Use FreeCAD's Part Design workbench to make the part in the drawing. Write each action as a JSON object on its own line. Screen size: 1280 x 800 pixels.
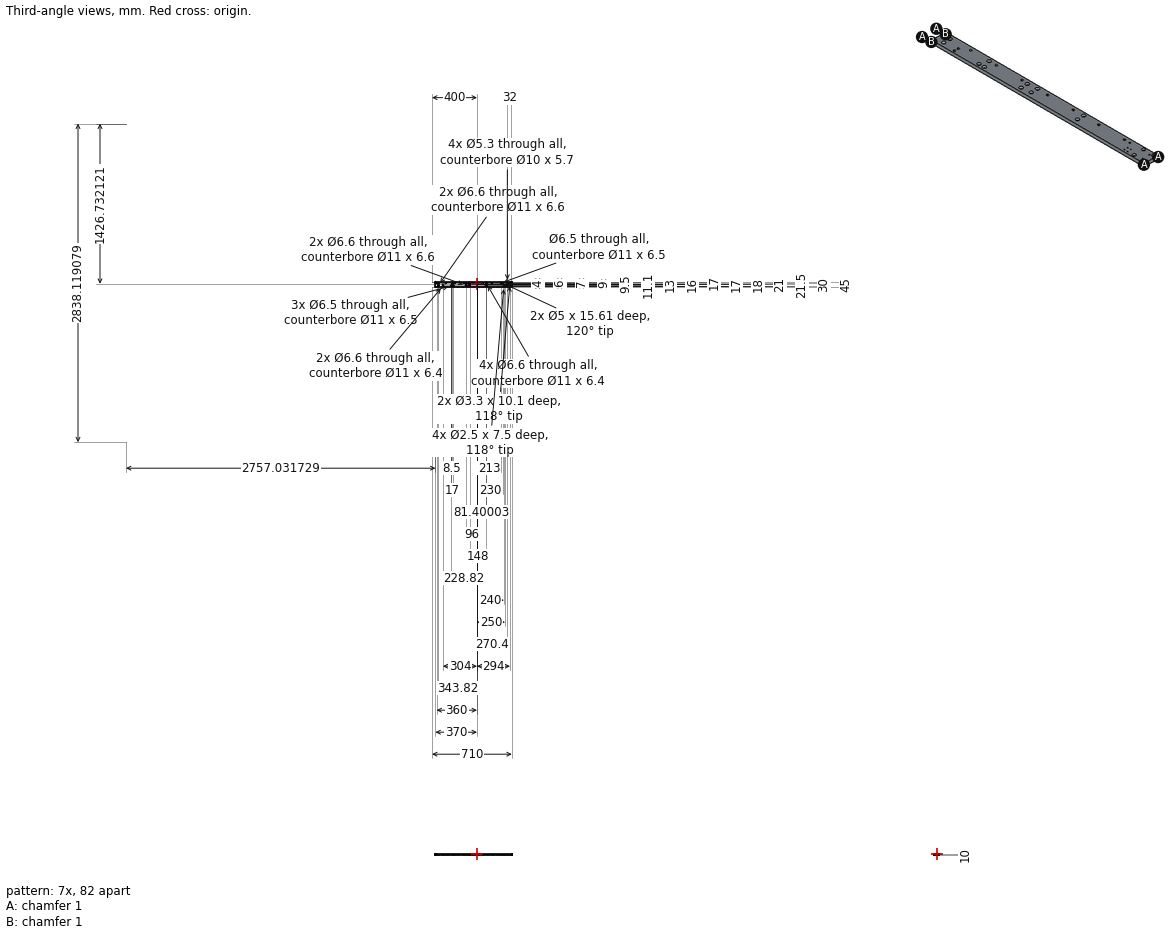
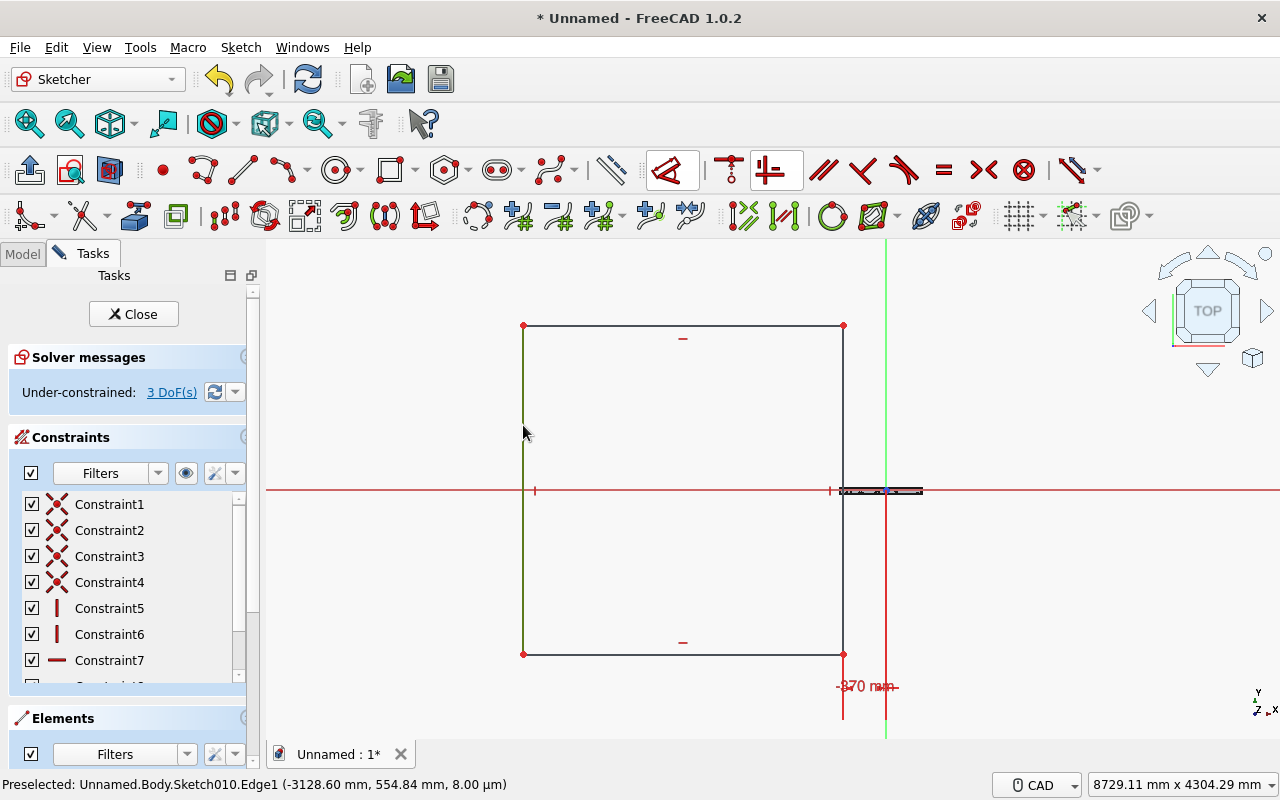
{"action": "left_click", "coordinate": [694, 170]}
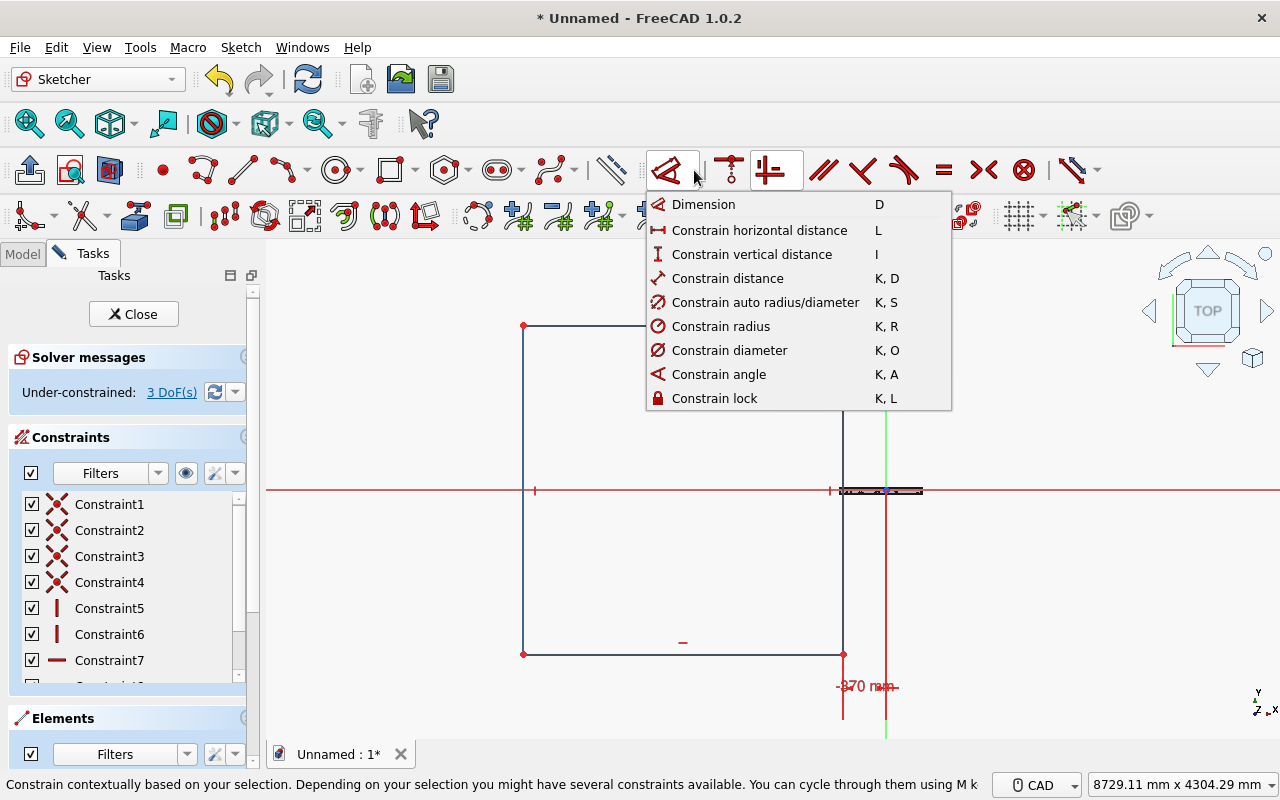
{"action": "left_click", "coordinate": [799, 254]}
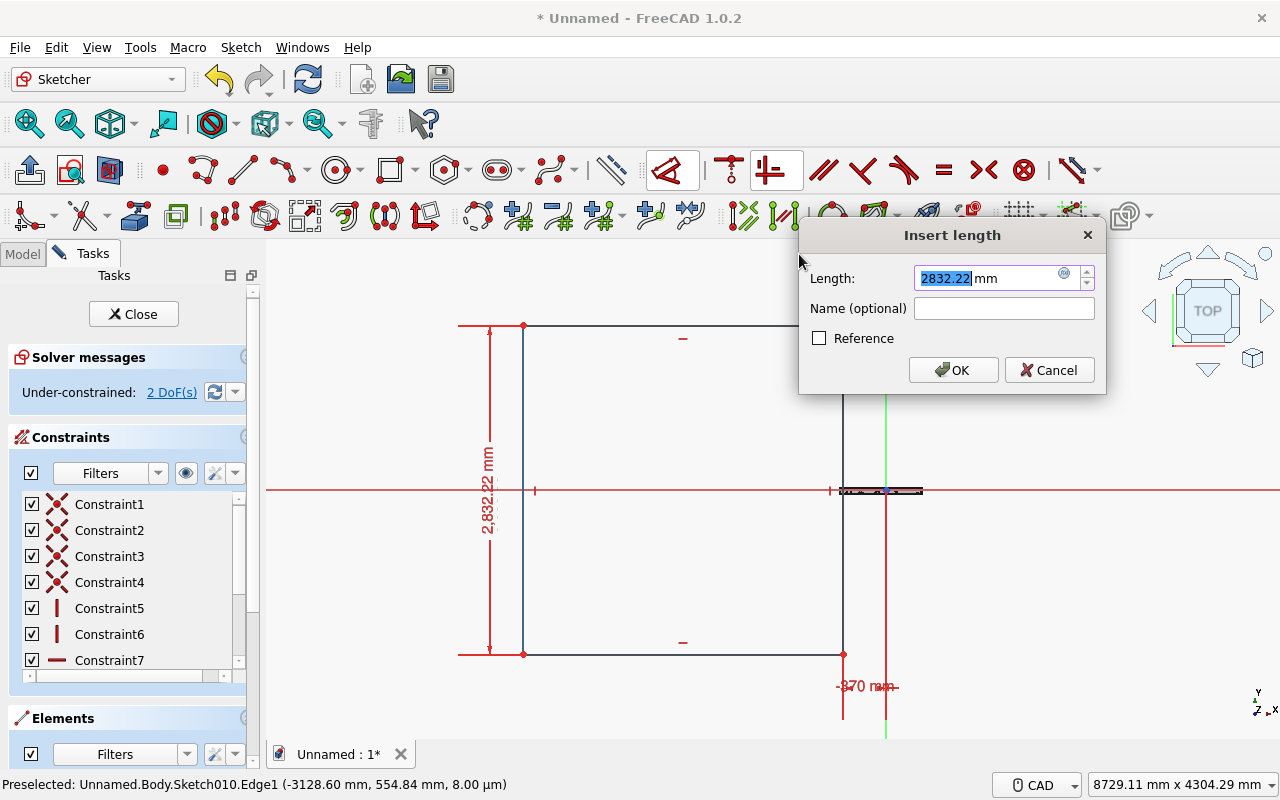
{"action": "type", "text": "2838.119079"}
{"action": "key", "text": "Return"}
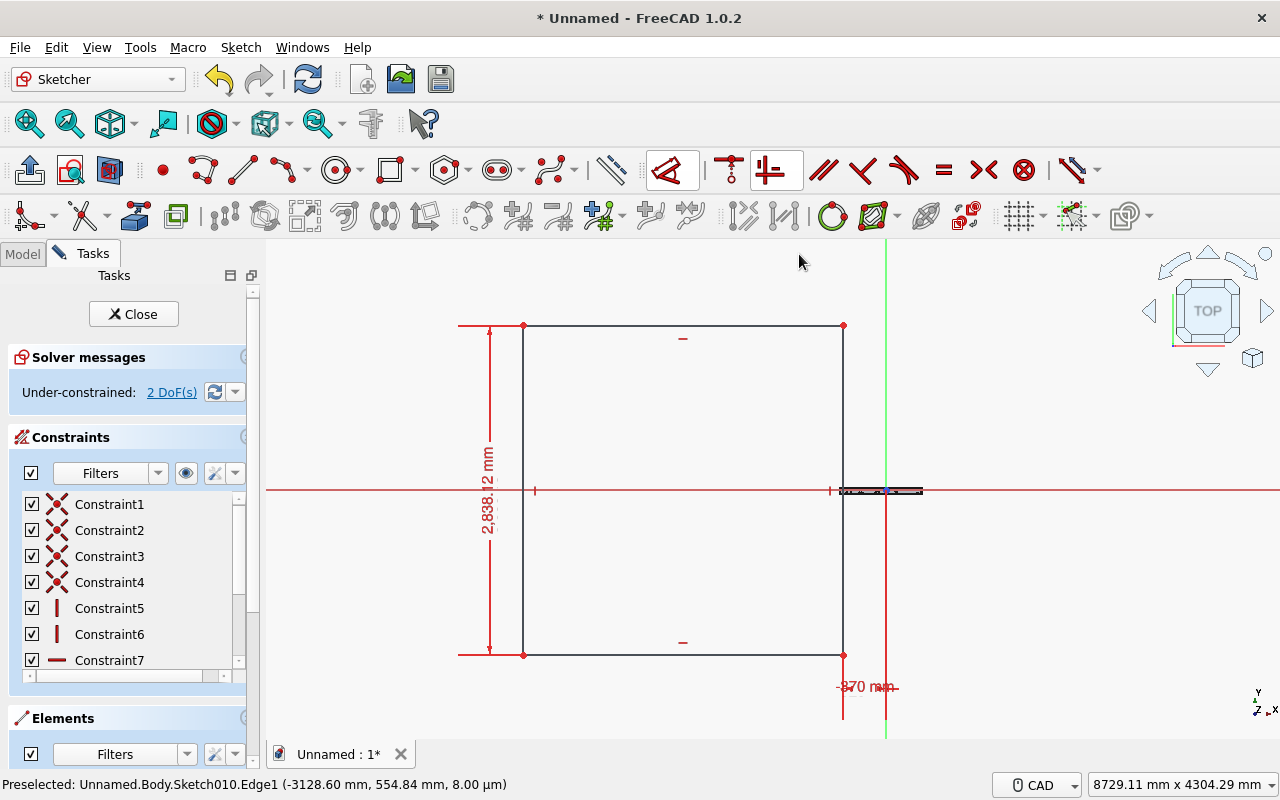
{"action": "left_click", "coordinate": [619, 655]}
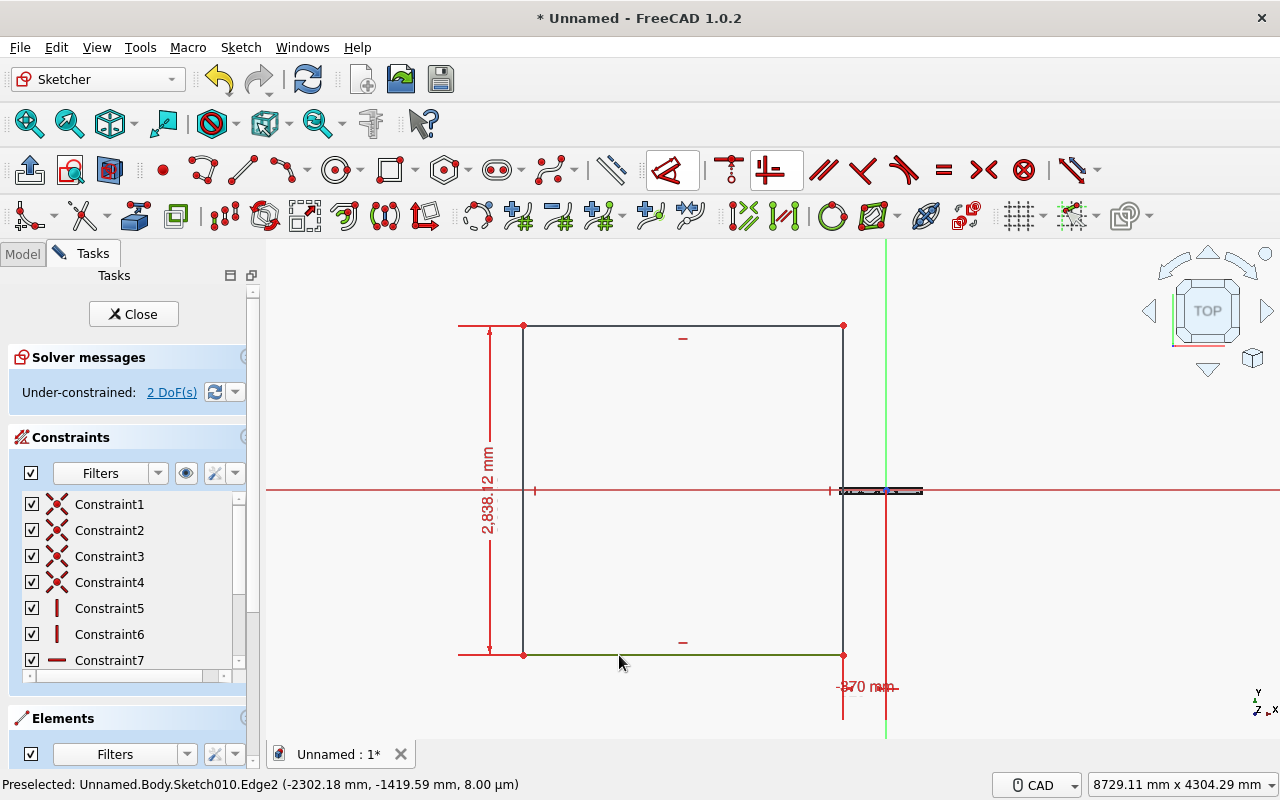
{"action": "left_click", "coordinate": [694, 170]}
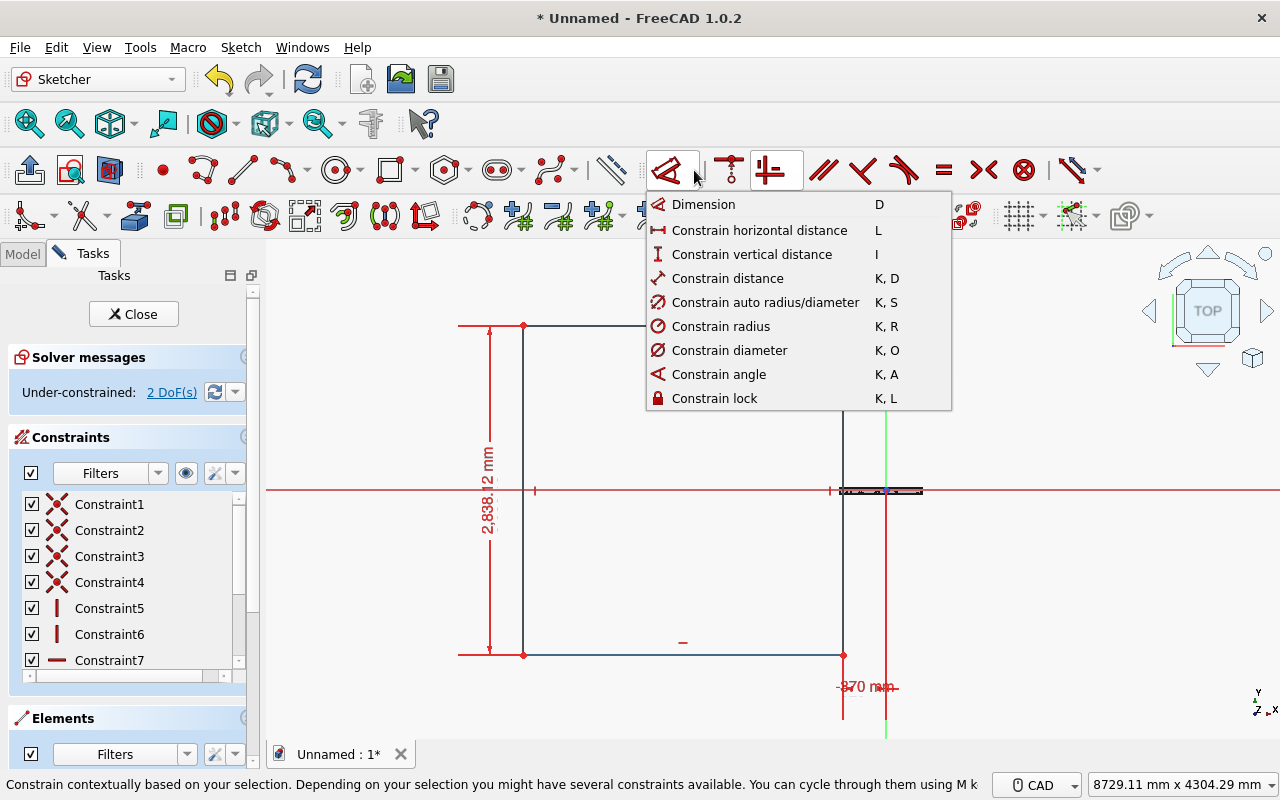
{"action": "left_click", "coordinate": [799, 230]}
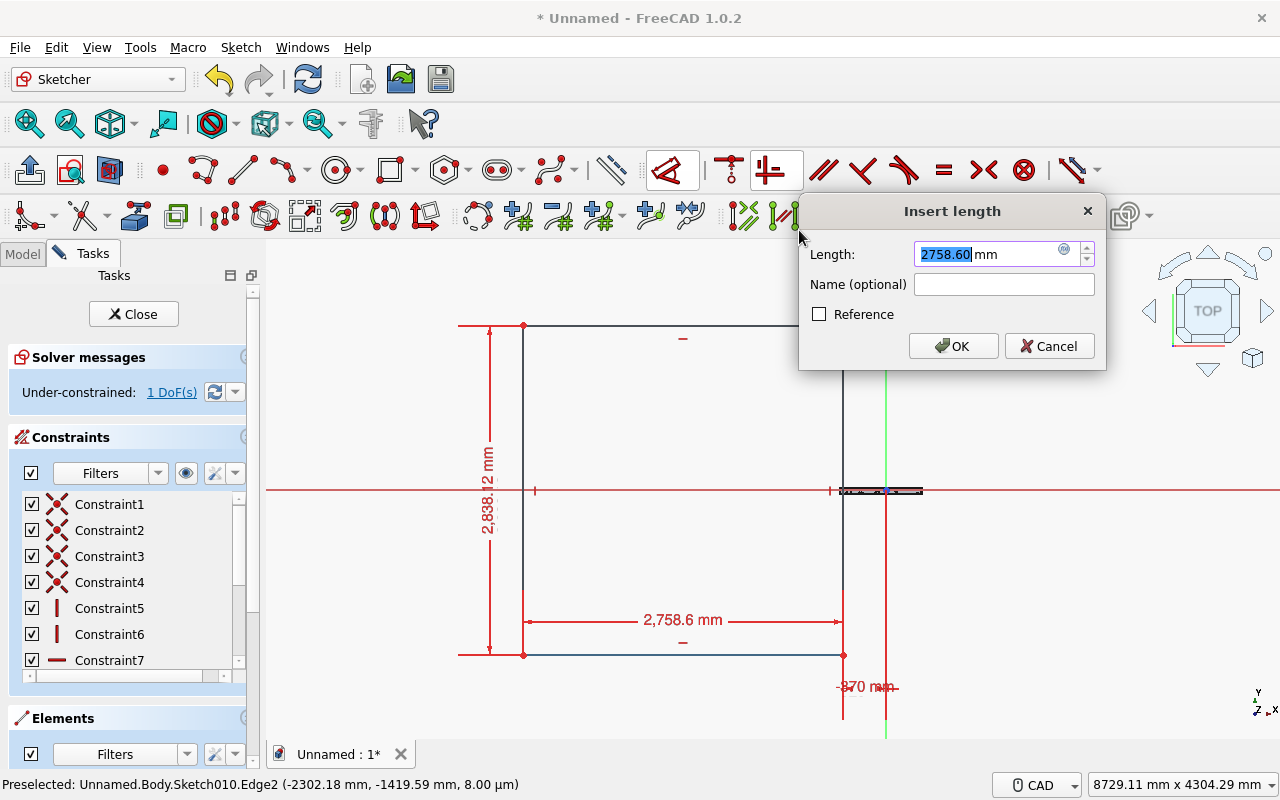
{"action": "type", "text": "2757.031729"}
{"action": "key", "text": "Return"}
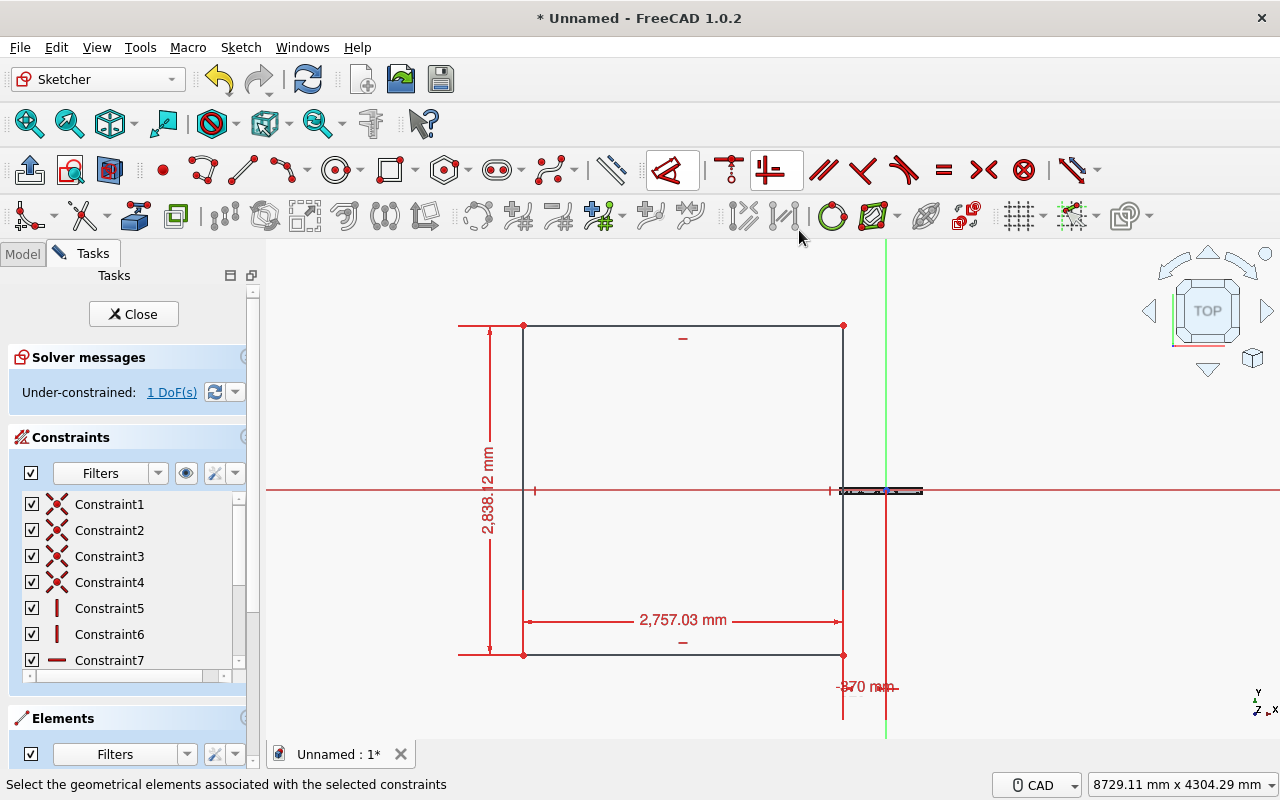
{"action": "left_click", "coordinate": [523, 326]}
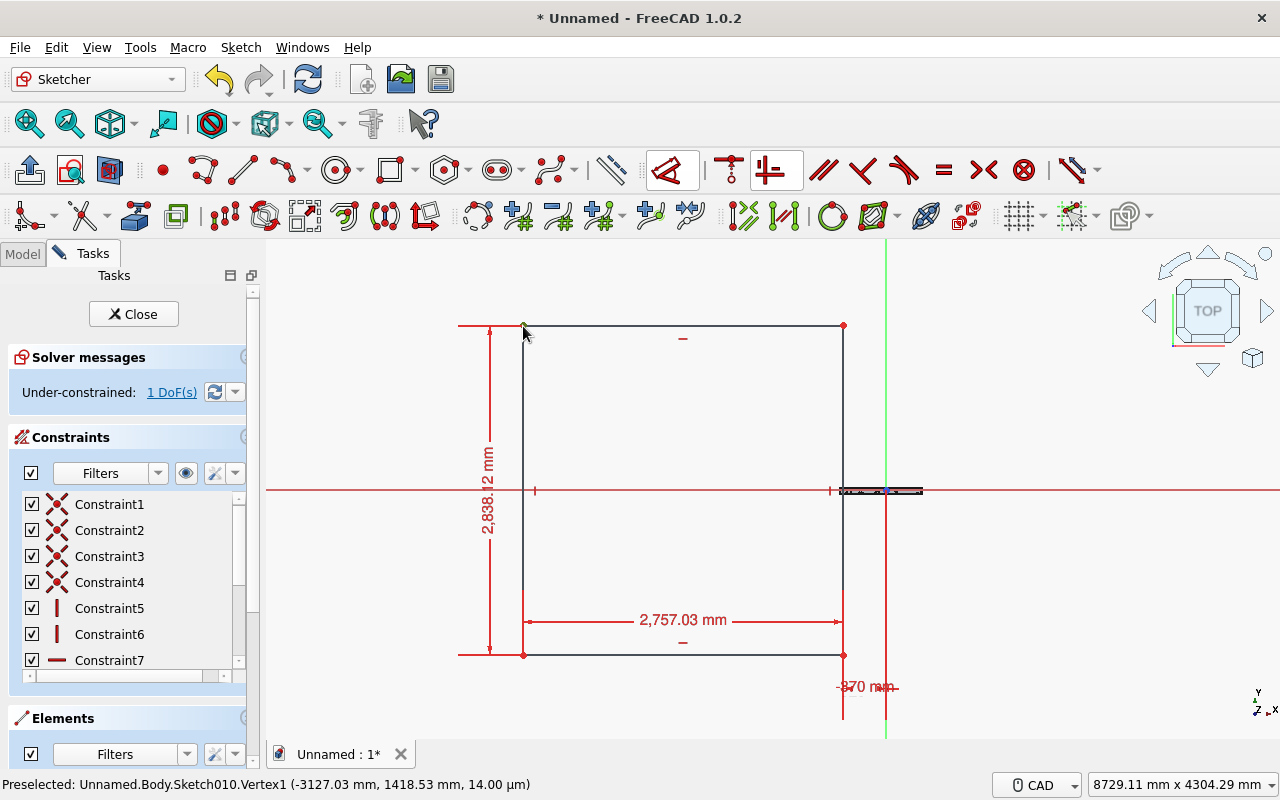
{"action": "left_click", "coordinate": [694, 170]}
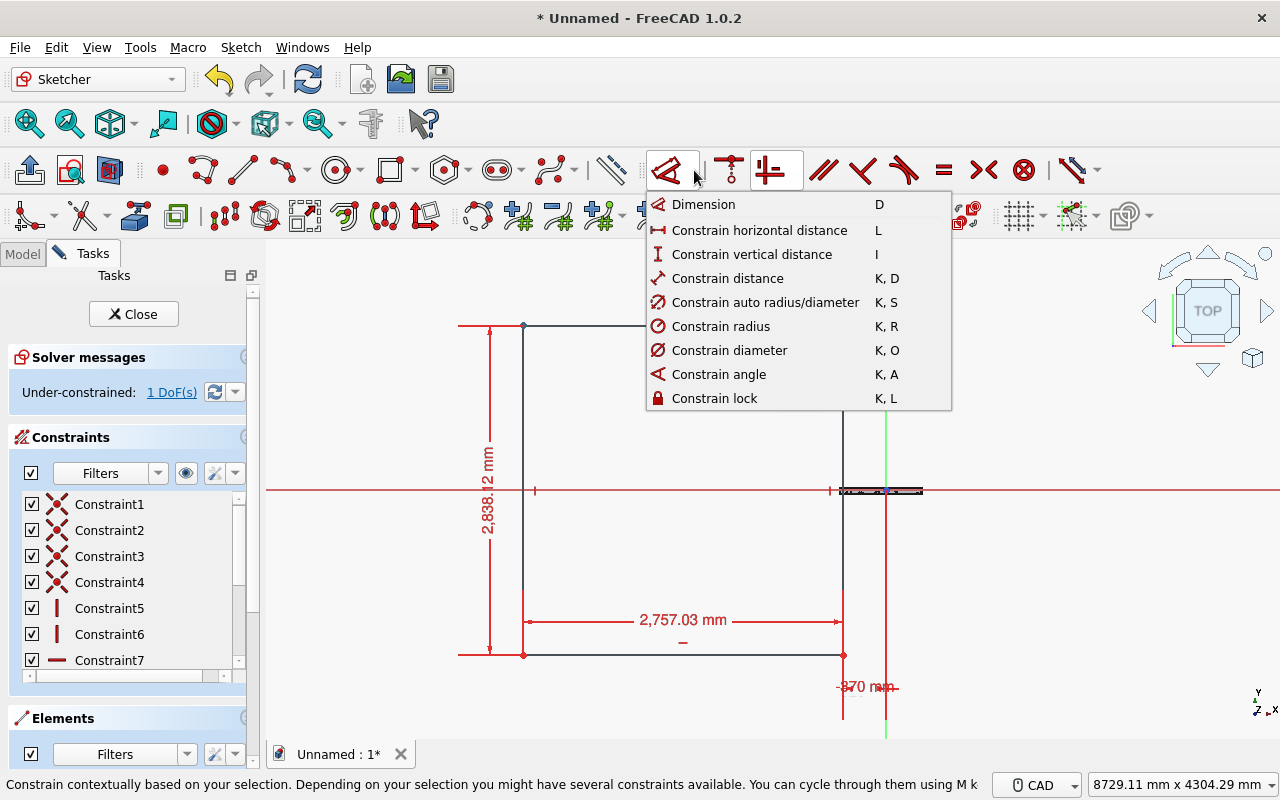
{"action": "left_click", "coordinate": [799, 254]}